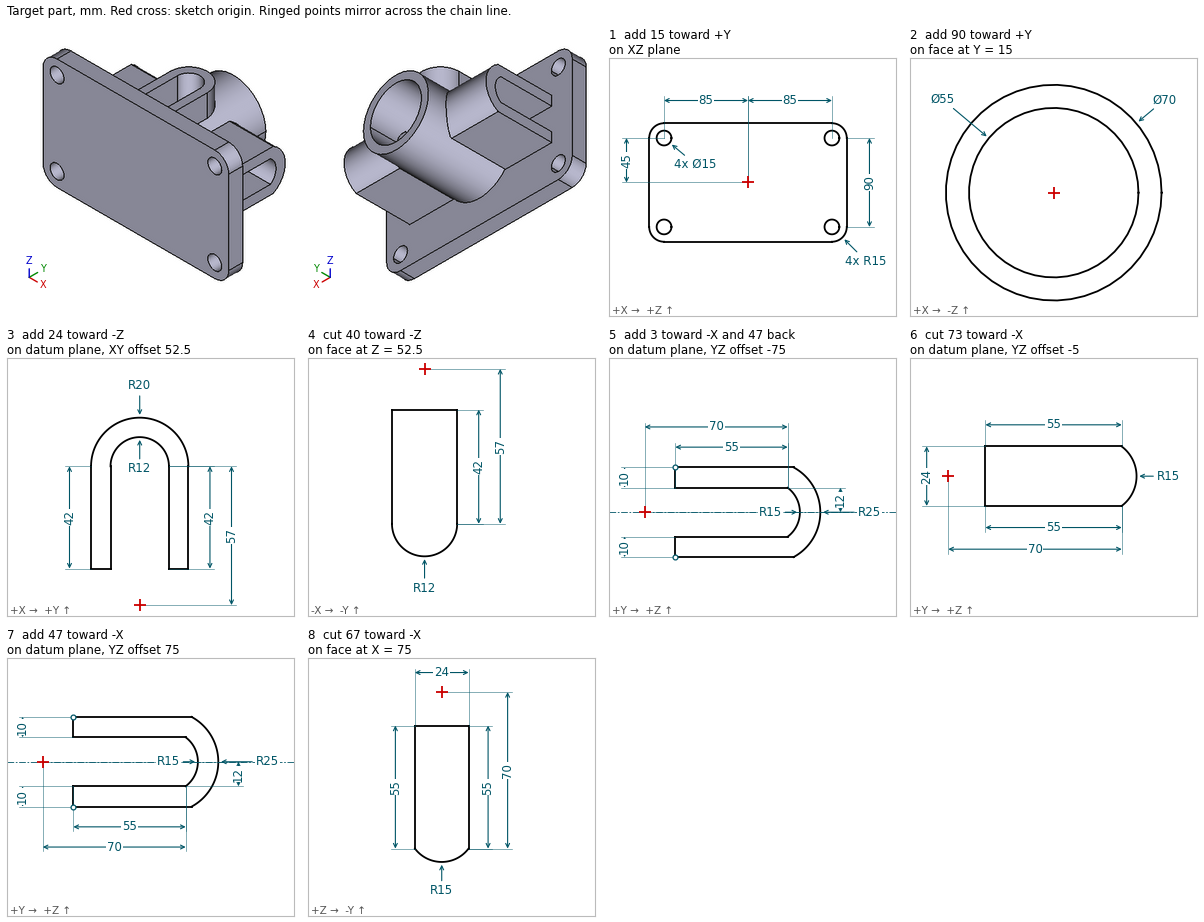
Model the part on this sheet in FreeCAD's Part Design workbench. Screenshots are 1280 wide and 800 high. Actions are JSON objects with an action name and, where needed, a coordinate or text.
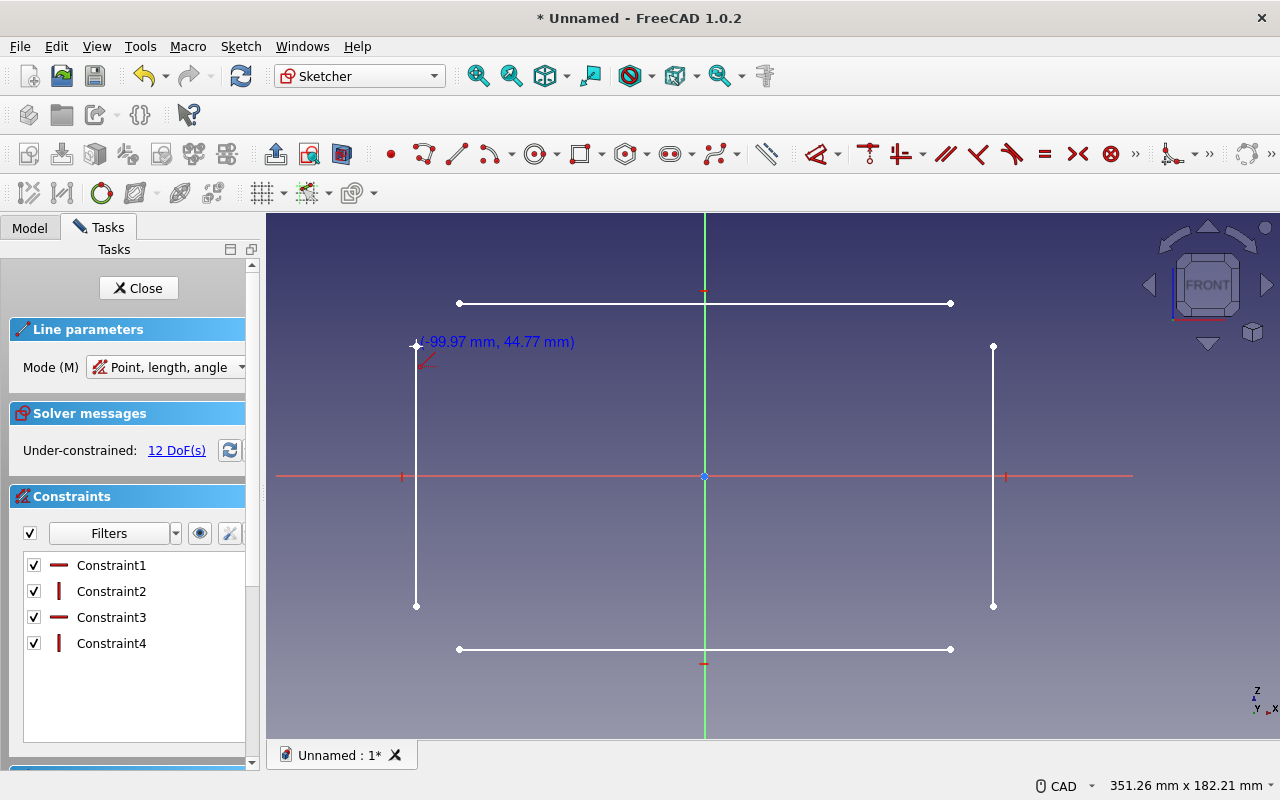
{"action": "key", "text": "g 3 a"}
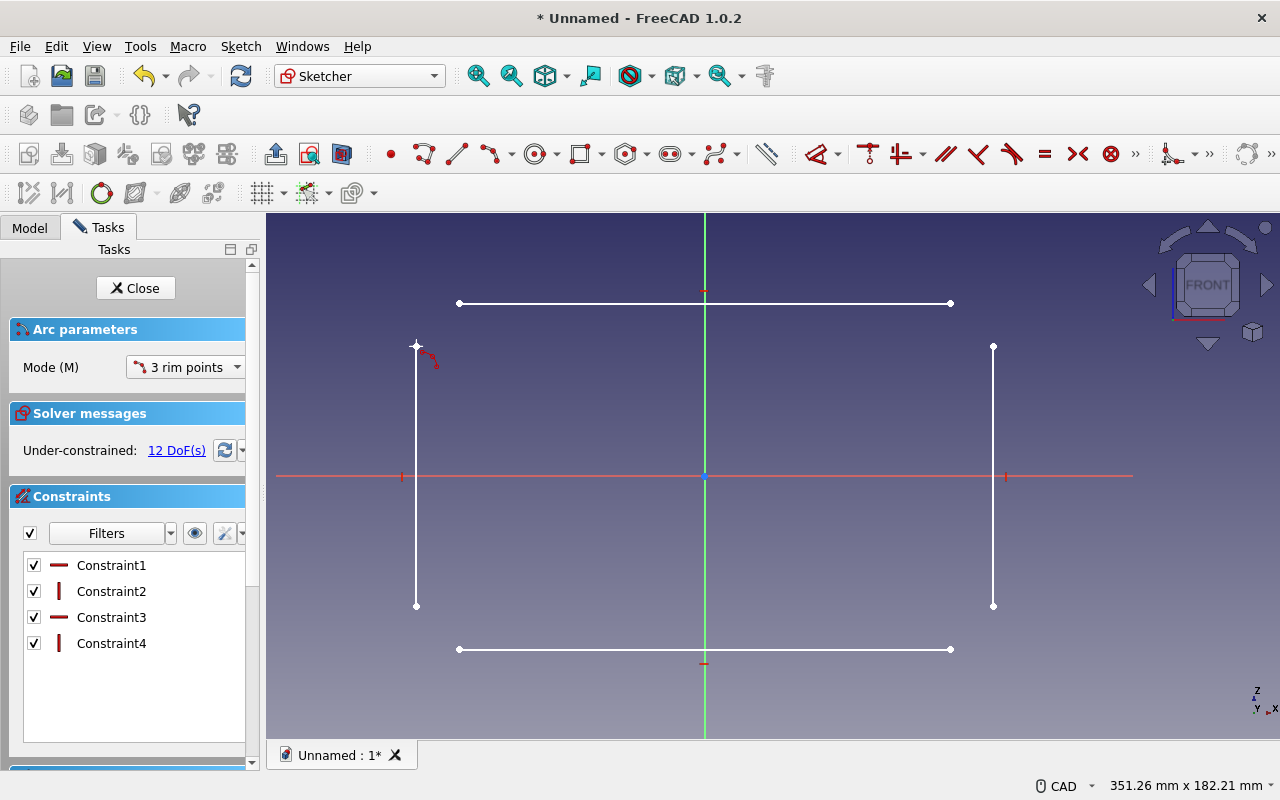
{"action": "left_click", "coordinate": [950, 304]}
{"action": "left_click", "coordinate": [993, 347]}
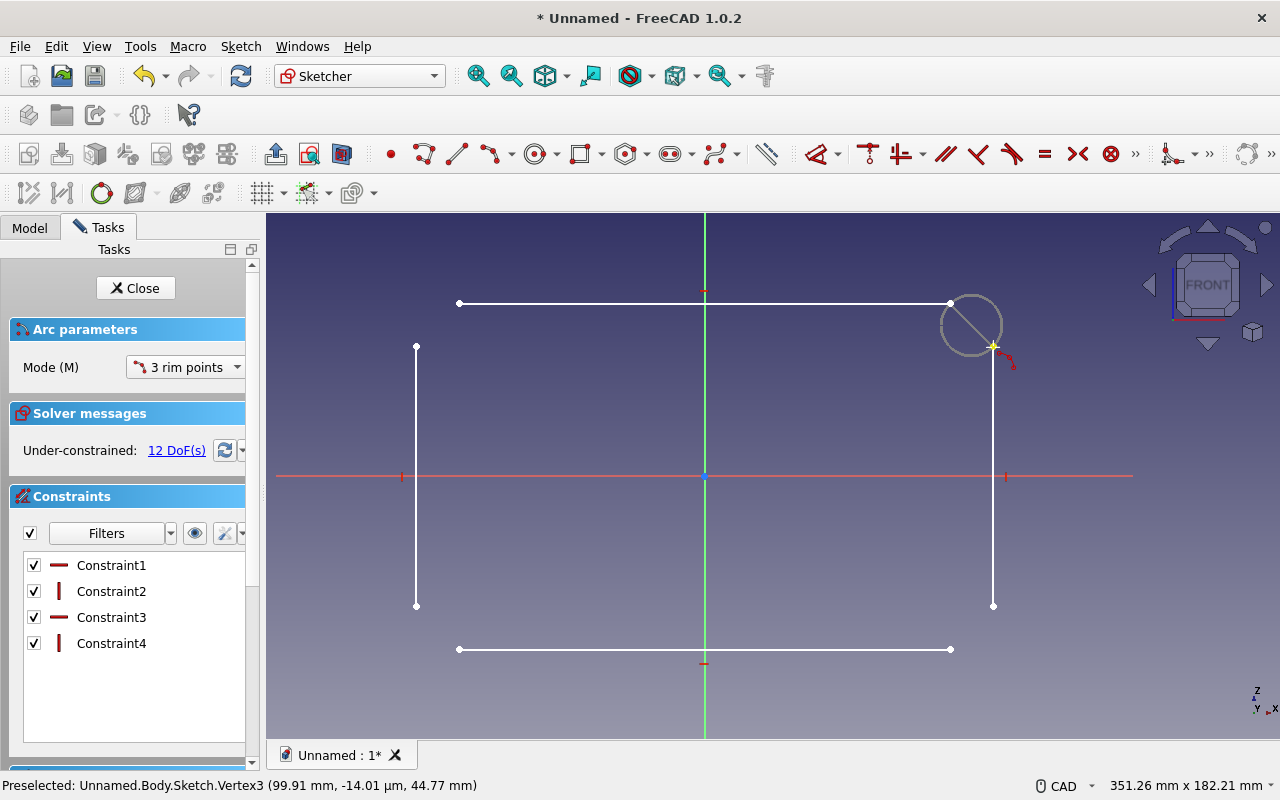
{"action": "scroll", "coordinate": [981, 316], "scroll_direction": "up", "scroll_amount": 2}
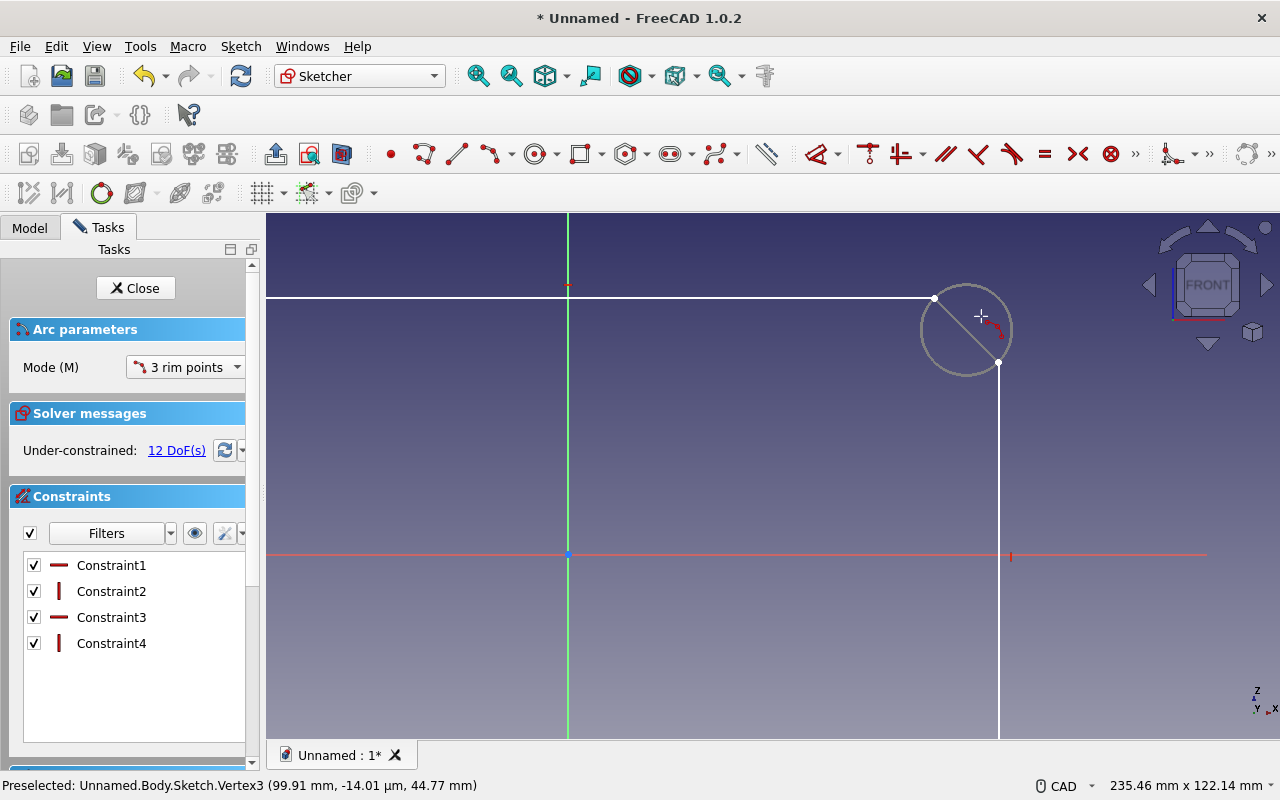
{"action": "left_click", "coordinate": [980, 315]}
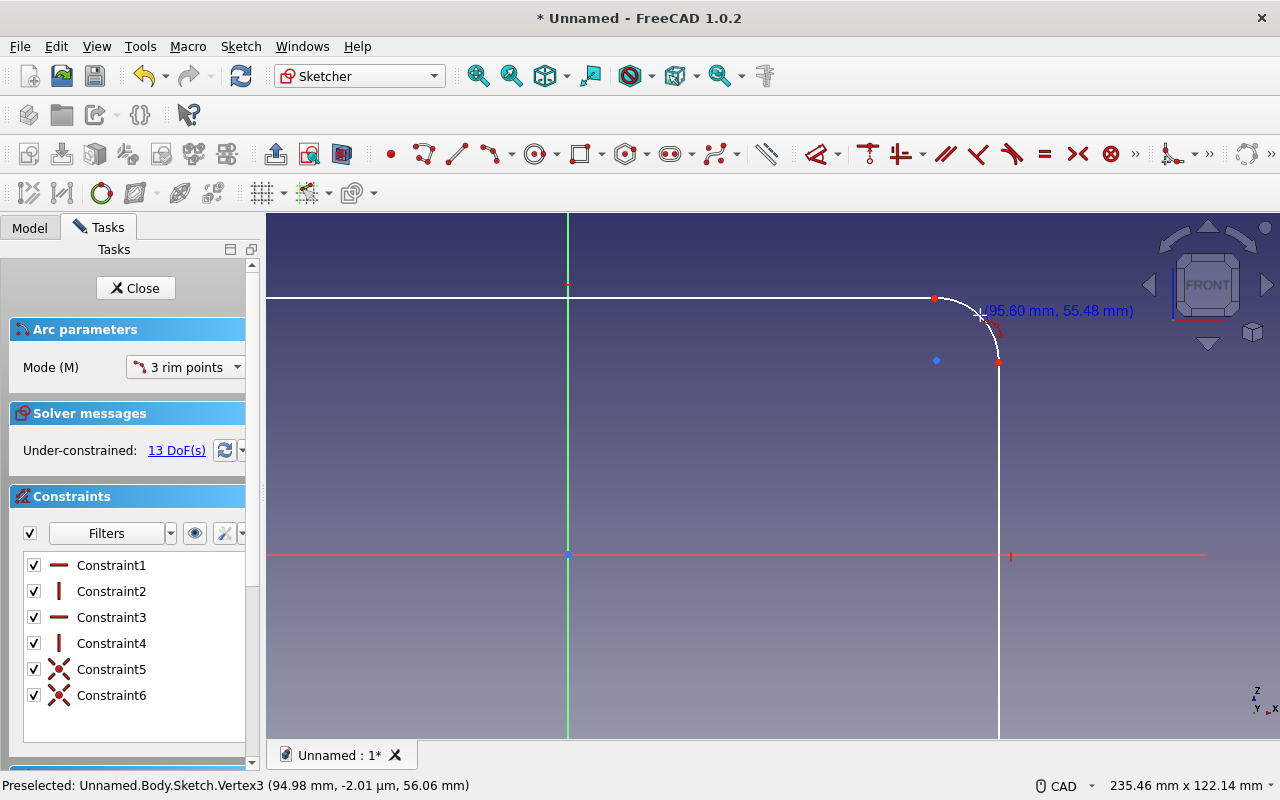
{"action": "scroll", "coordinate": [981, 316], "scroll_direction": "down", "scroll_amount": 2}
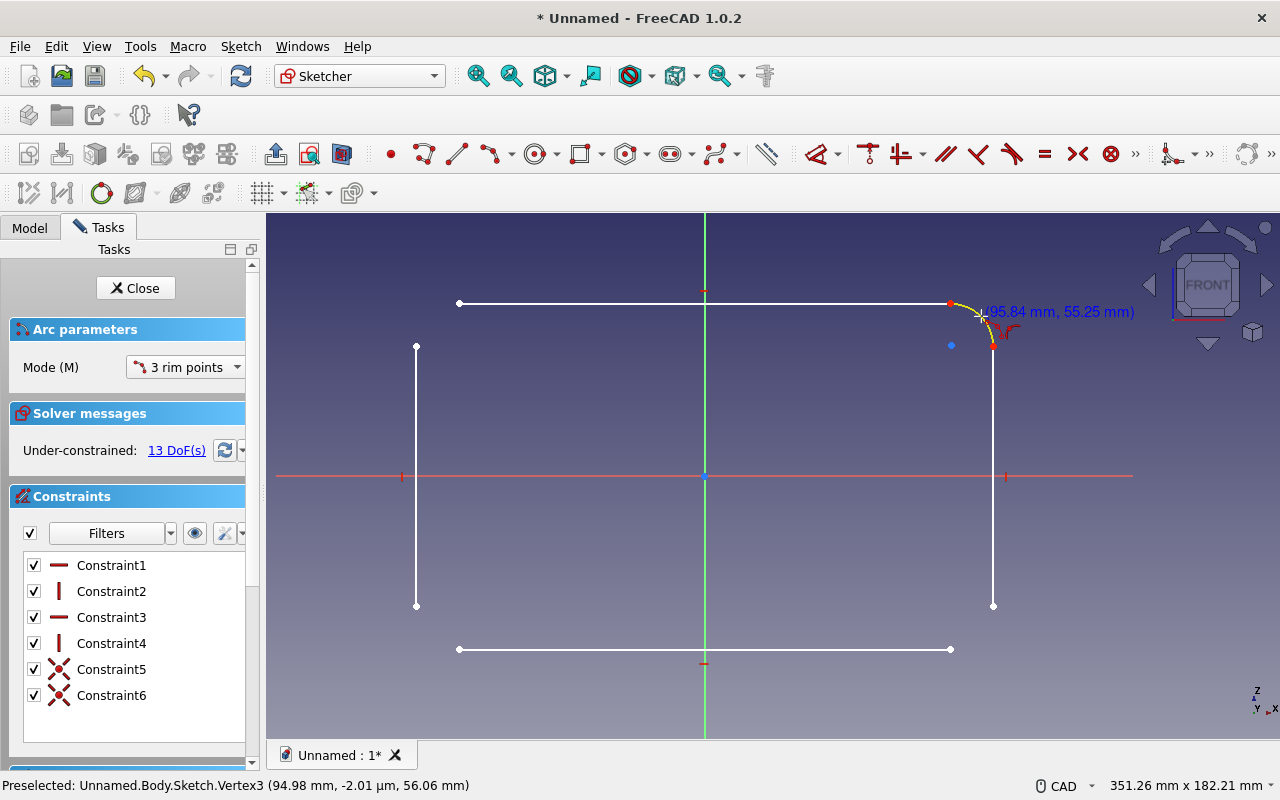
{"action": "left_click", "coordinate": [993, 607]}
{"action": "left_click", "coordinate": [950, 650]}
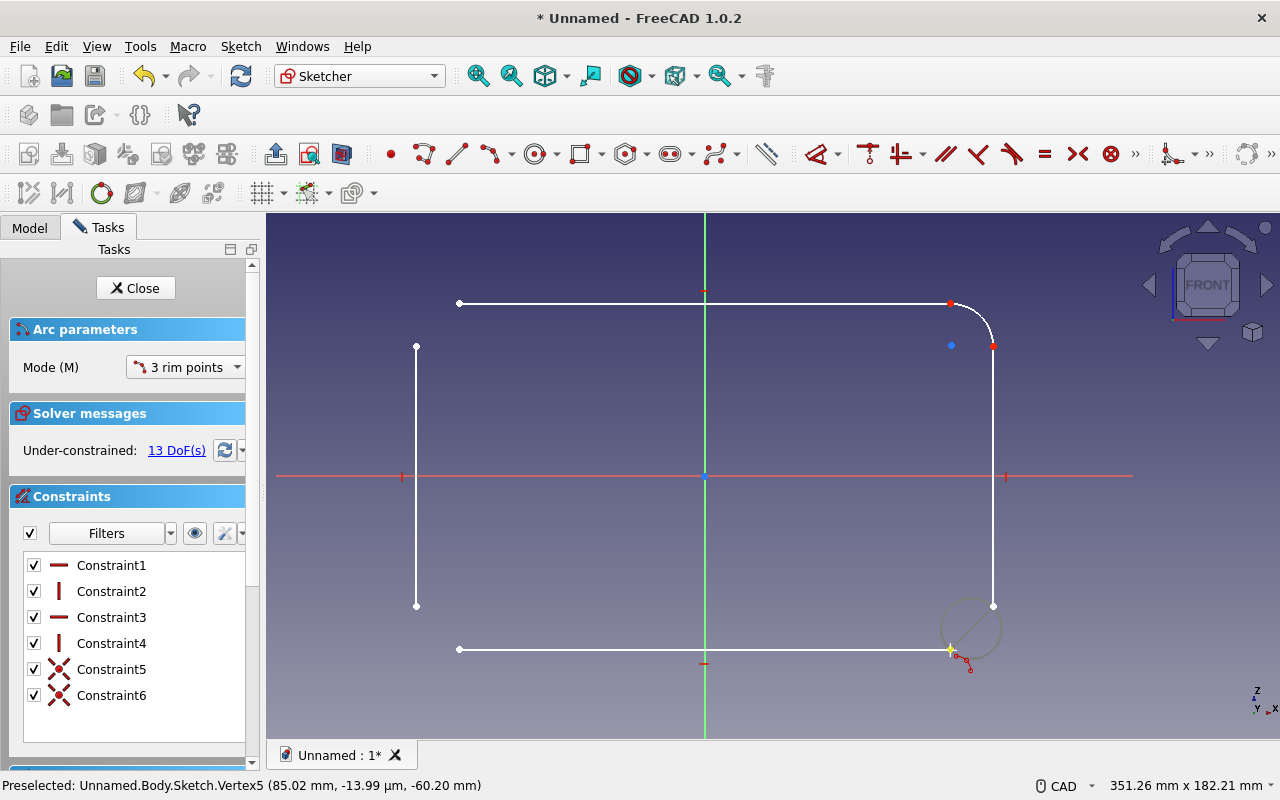
{"action": "scroll", "coordinate": [981, 637], "scroll_direction": "up", "scroll_amount": 2}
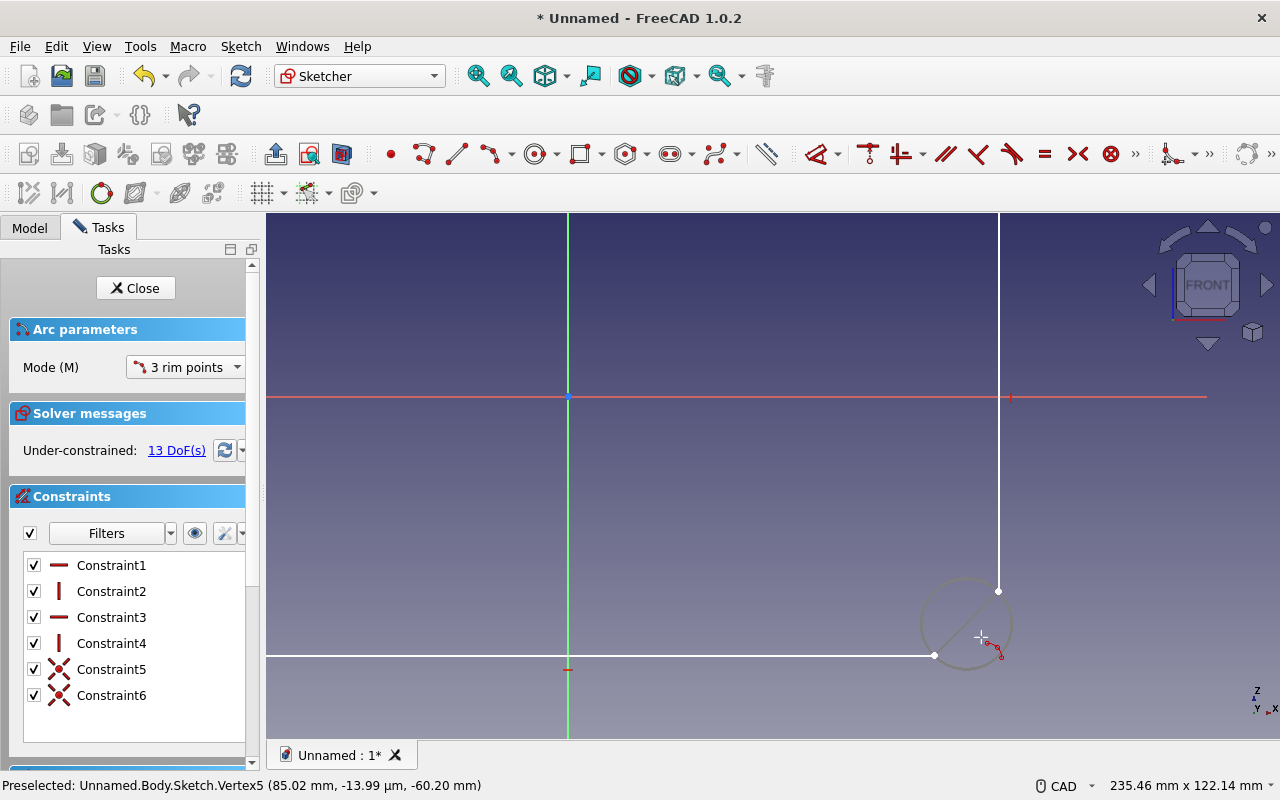
{"action": "left_click", "coordinate": [980, 636]}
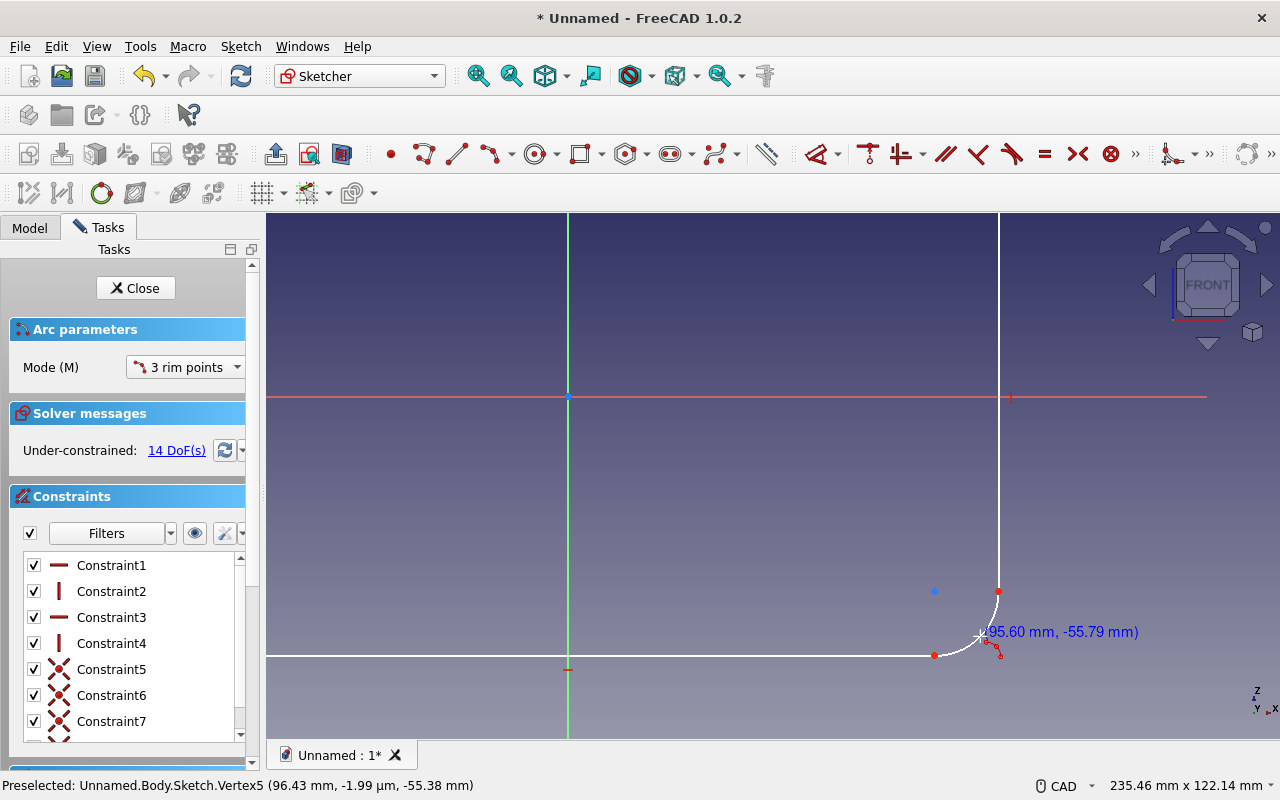
{"action": "scroll", "coordinate": [981, 637], "scroll_direction": "down", "scroll_amount": 2}